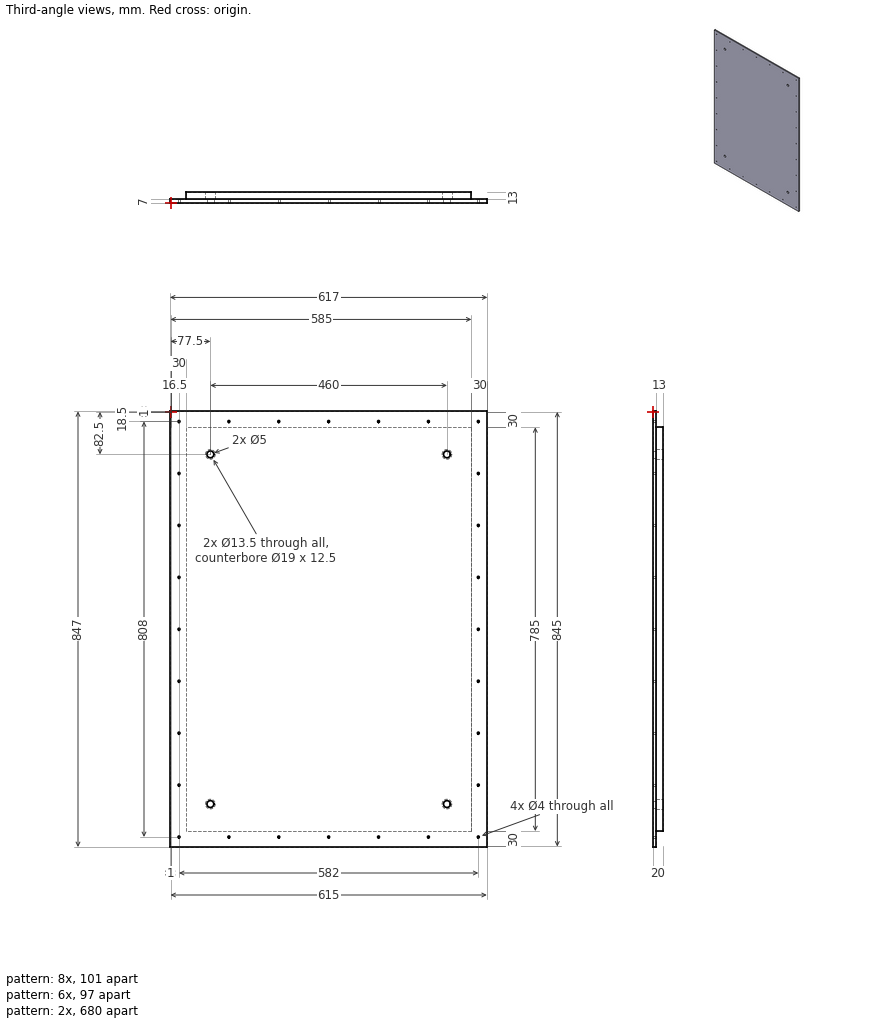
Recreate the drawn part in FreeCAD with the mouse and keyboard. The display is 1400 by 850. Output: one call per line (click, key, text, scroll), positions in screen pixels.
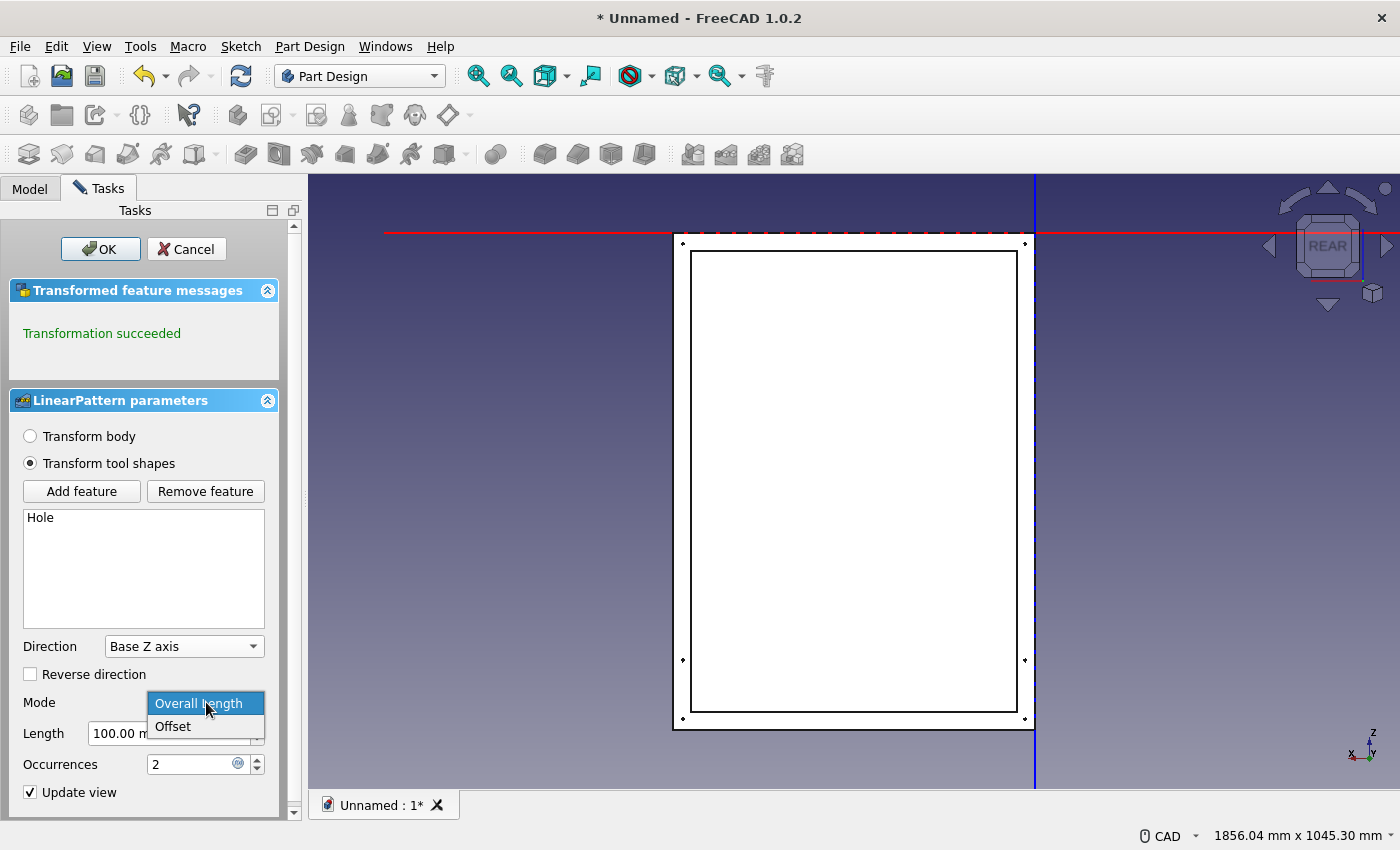
click(204, 726)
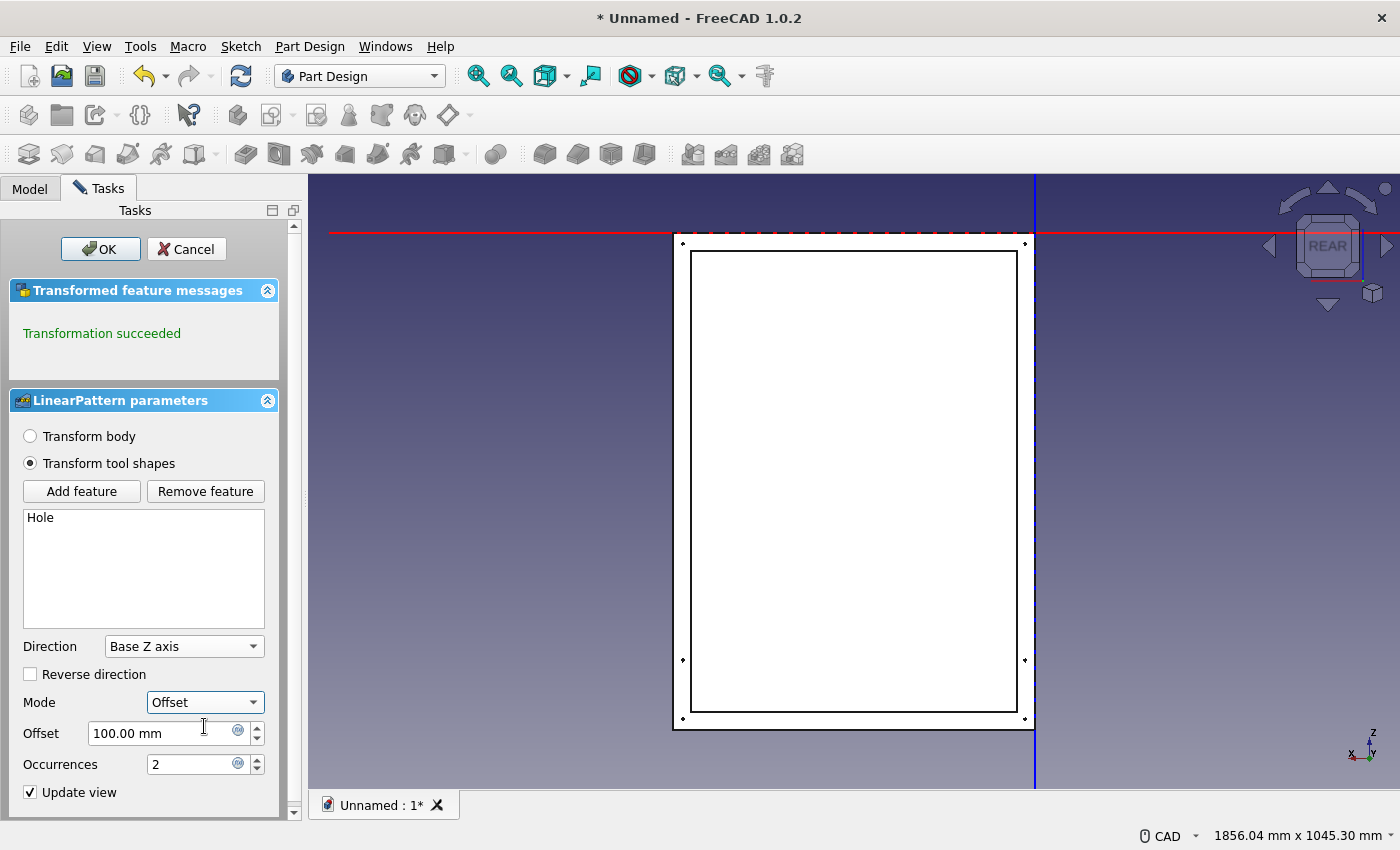
triple_click(170, 734)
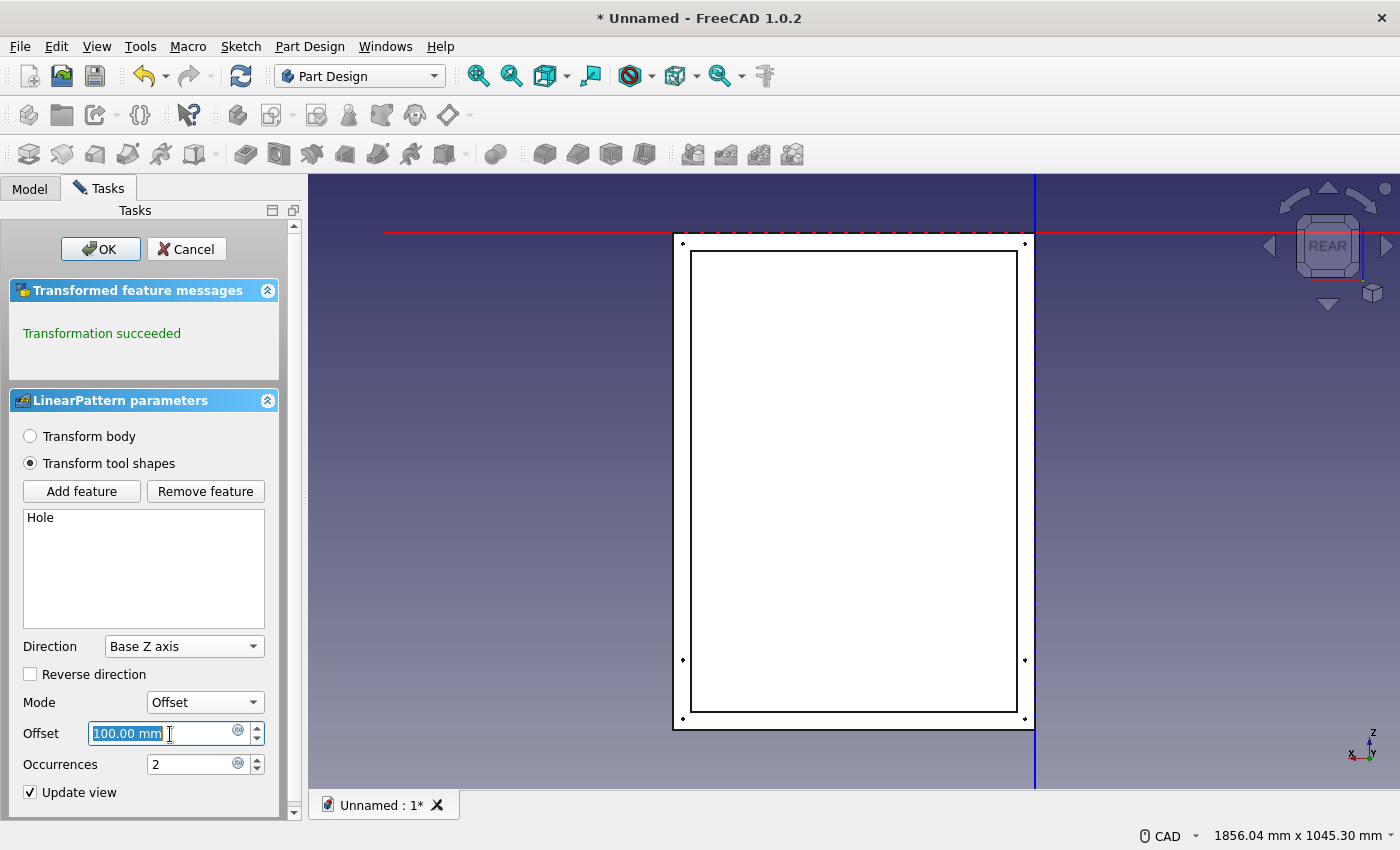
text(101)
key(Tab)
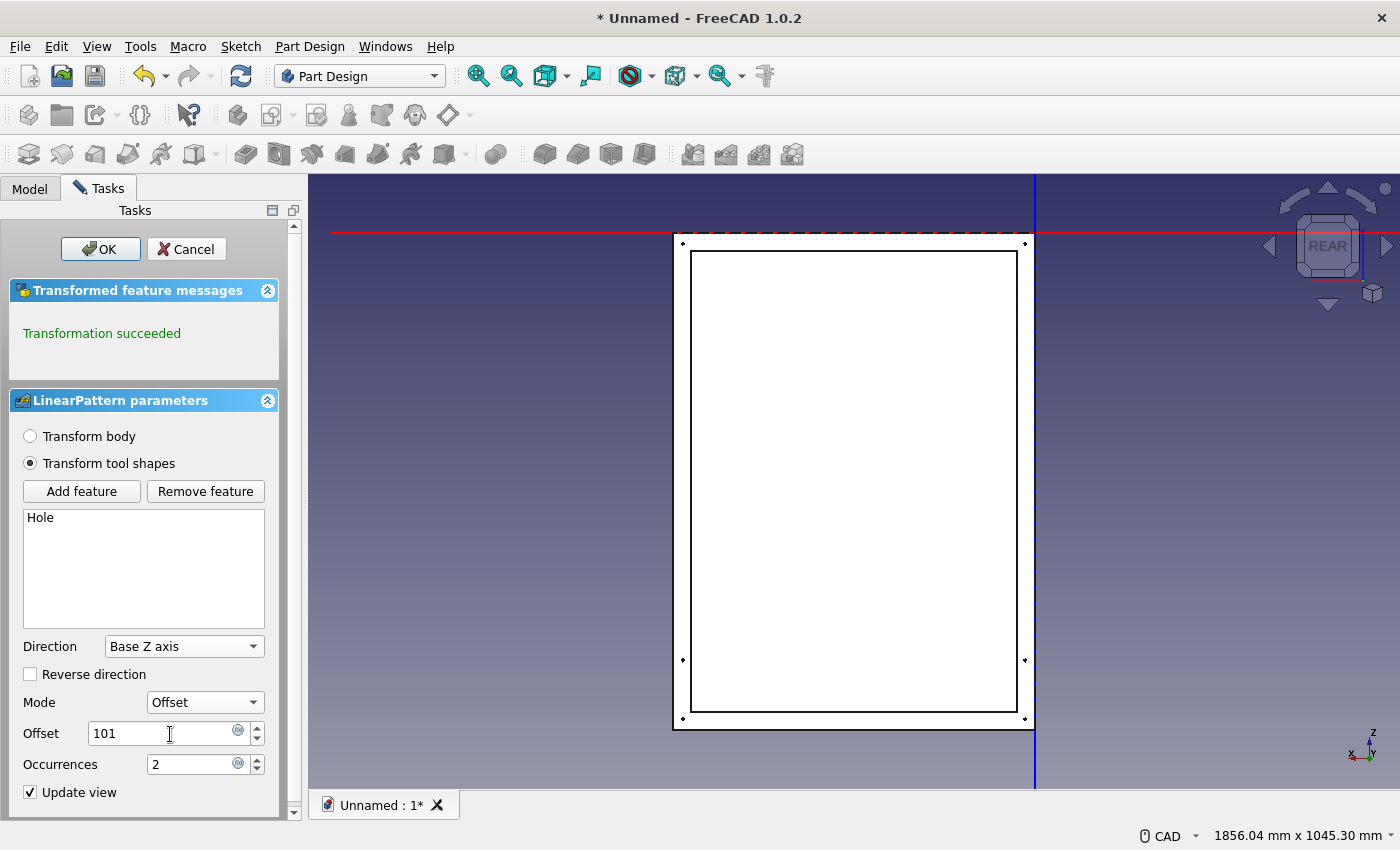
triple_click(199, 764)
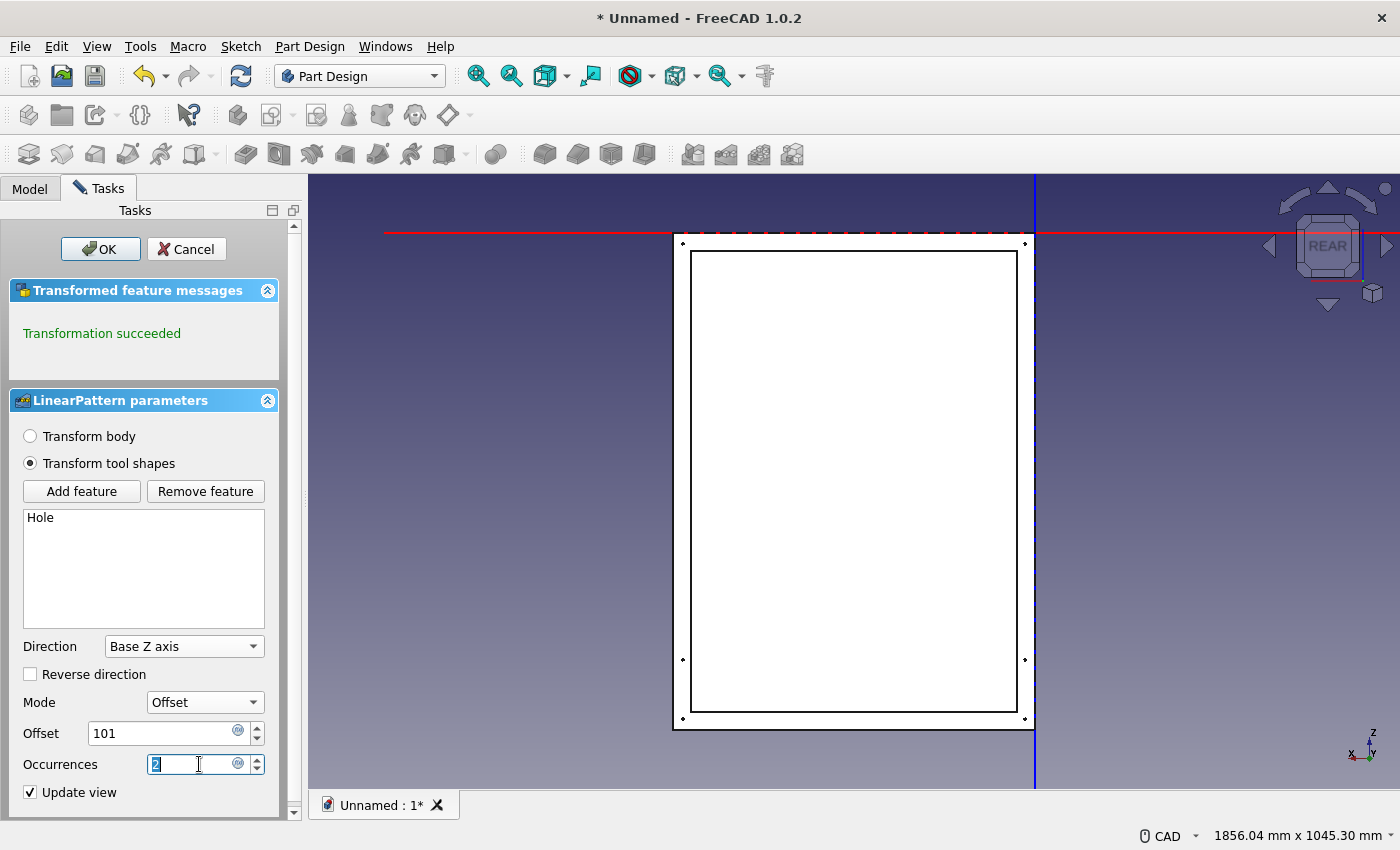
text(8)
key(Tab)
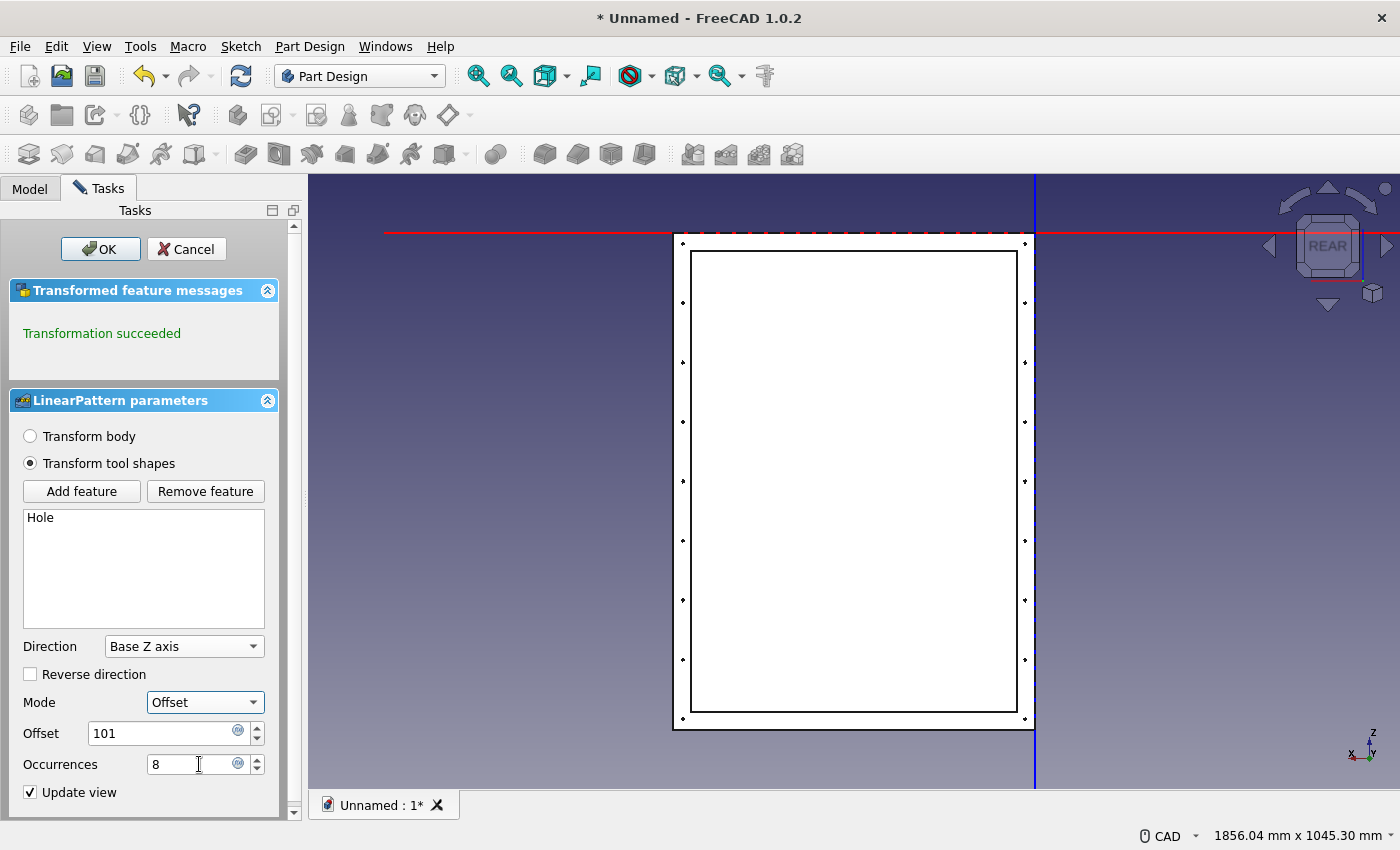
click(101, 249)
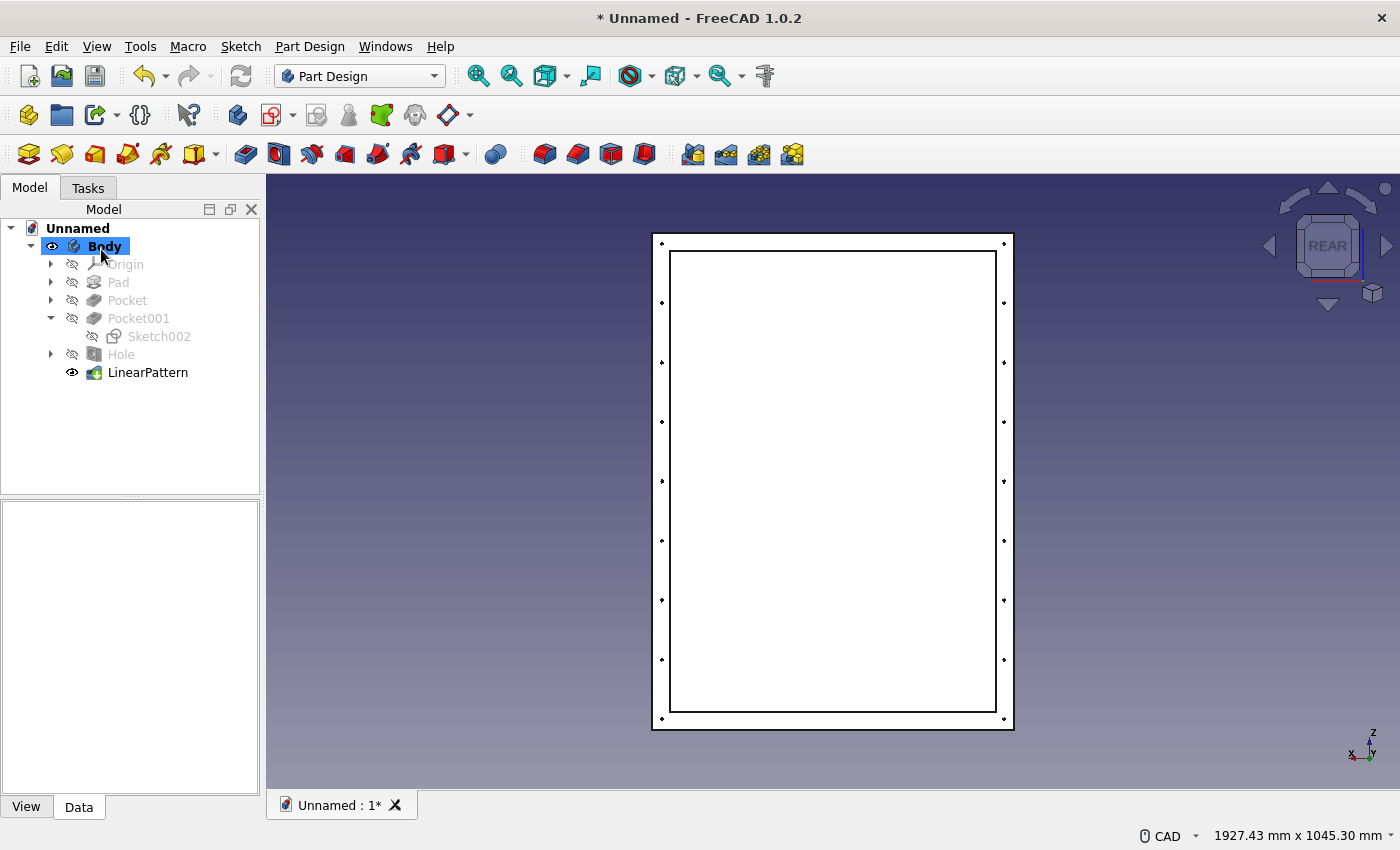
click(117, 354)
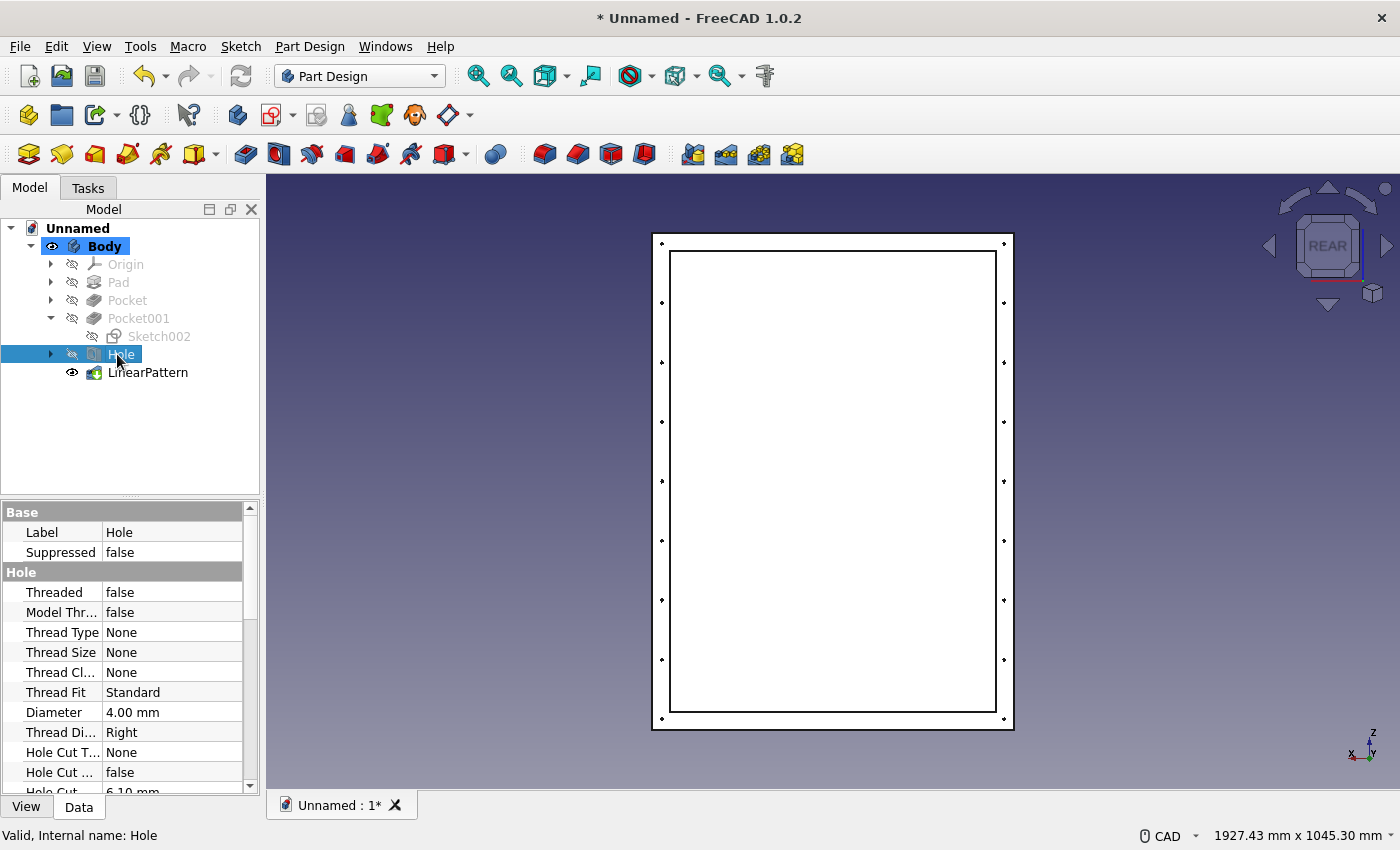
click(726, 154)